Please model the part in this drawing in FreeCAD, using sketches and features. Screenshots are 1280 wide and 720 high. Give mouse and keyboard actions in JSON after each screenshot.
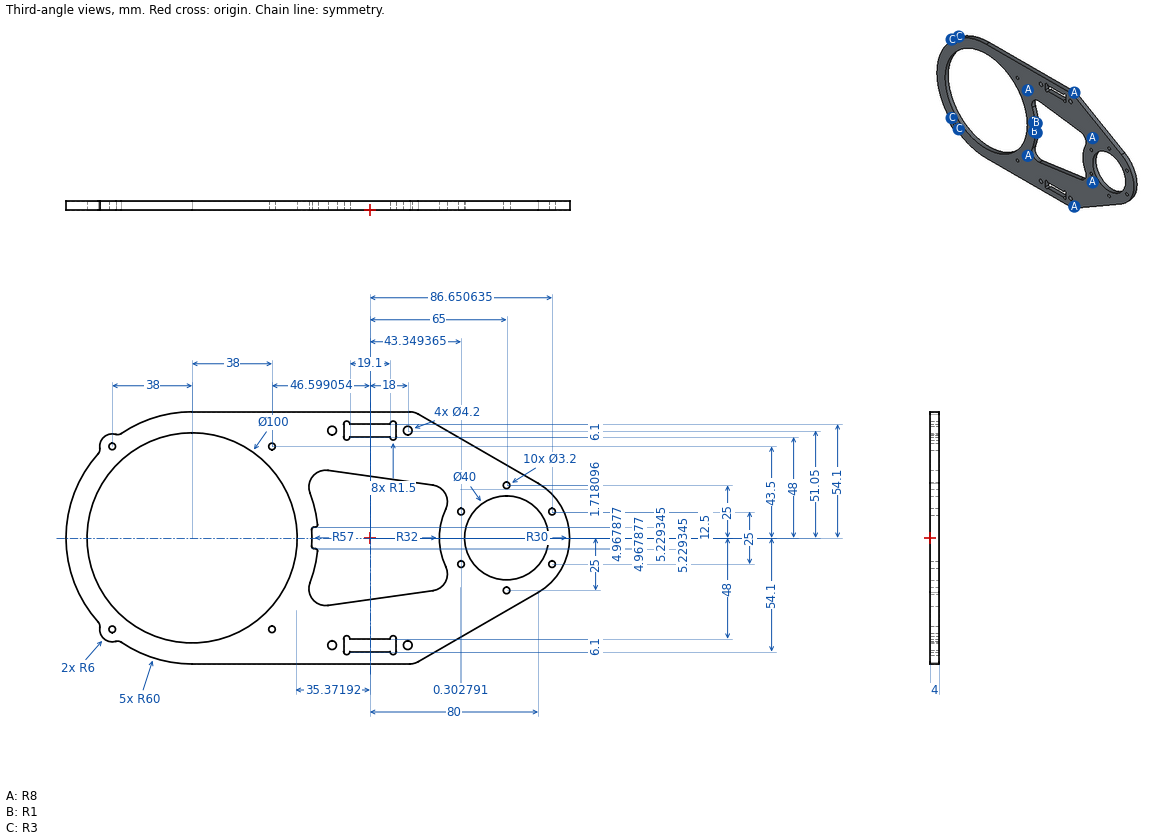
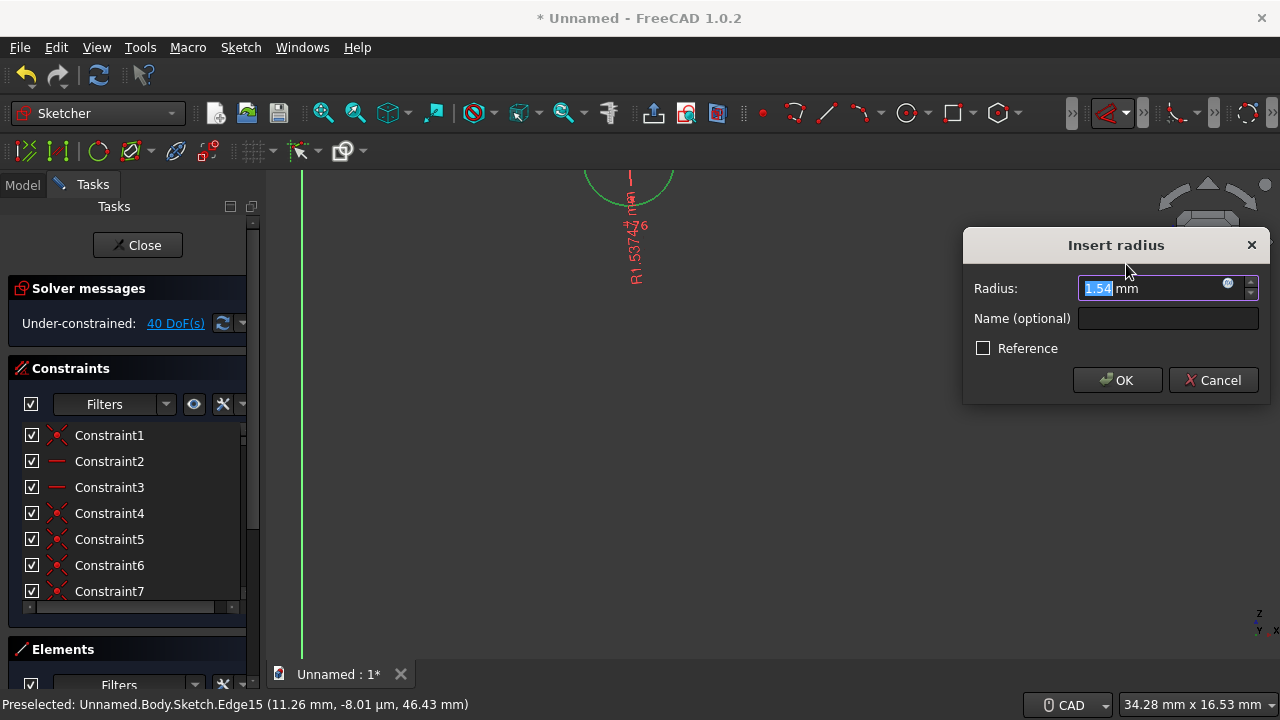
{"action": "type", "text": "1.5"}
{"action": "key", "text": "Return"}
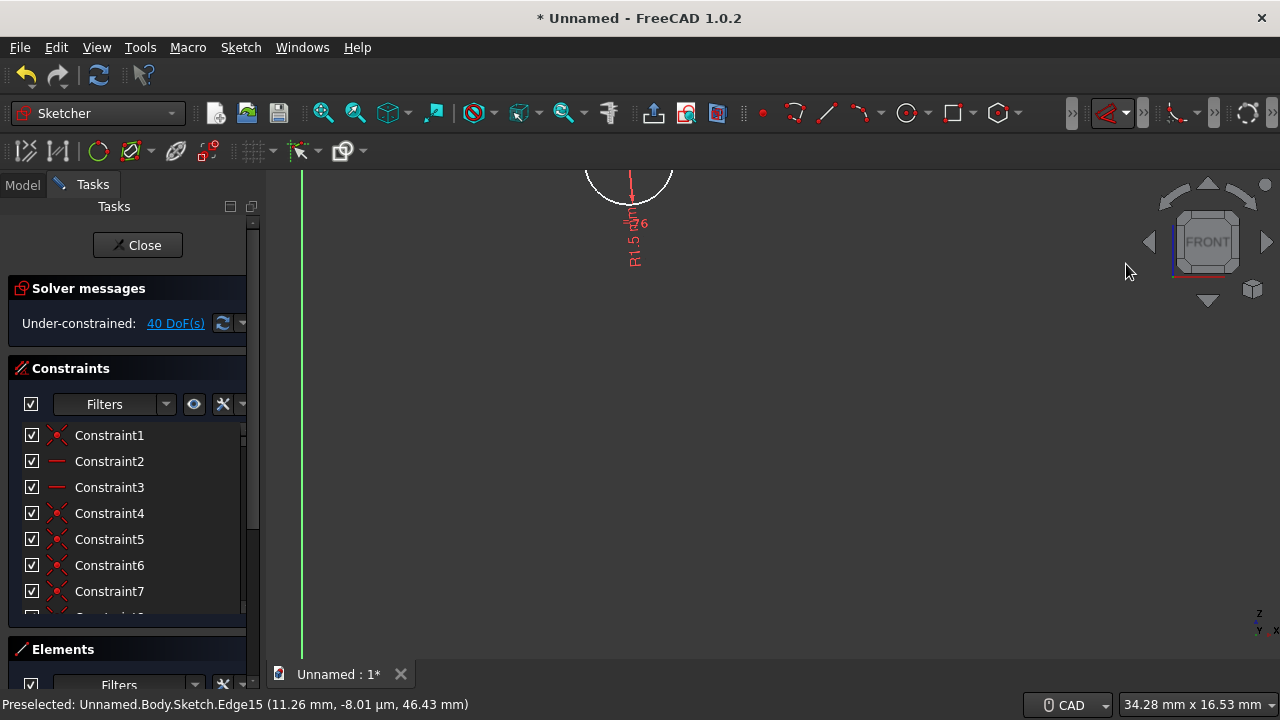
{"action": "scroll", "coordinate": [796, 321], "scroll_direction": "down", "scroll_amount": 13}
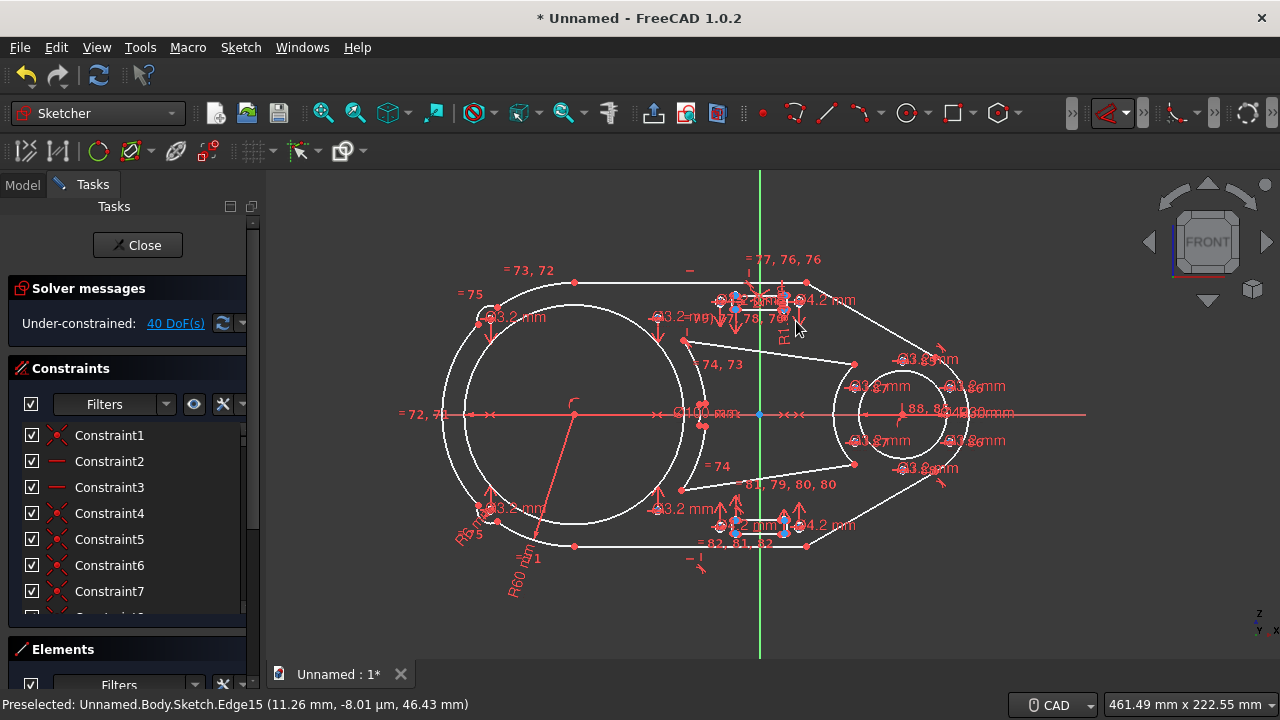
{"action": "left_click", "coordinate": [837, 393]}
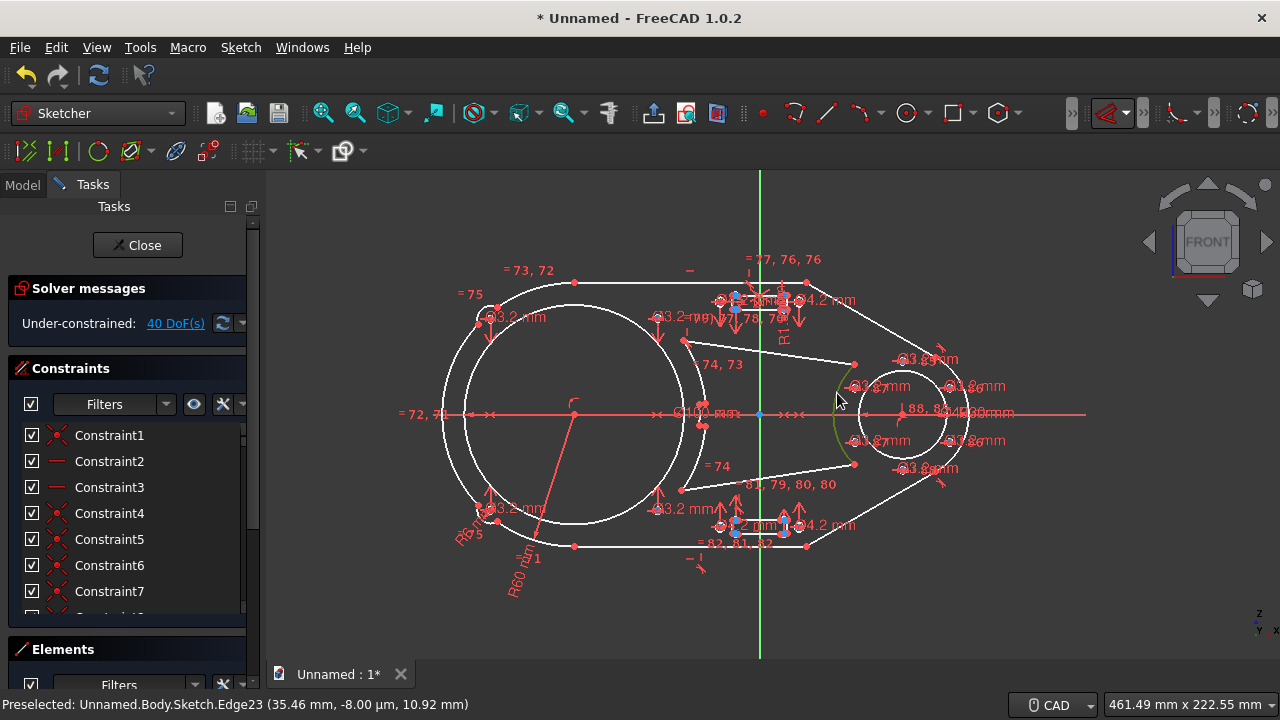
{"action": "left_click", "coordinate": [1128, 114]}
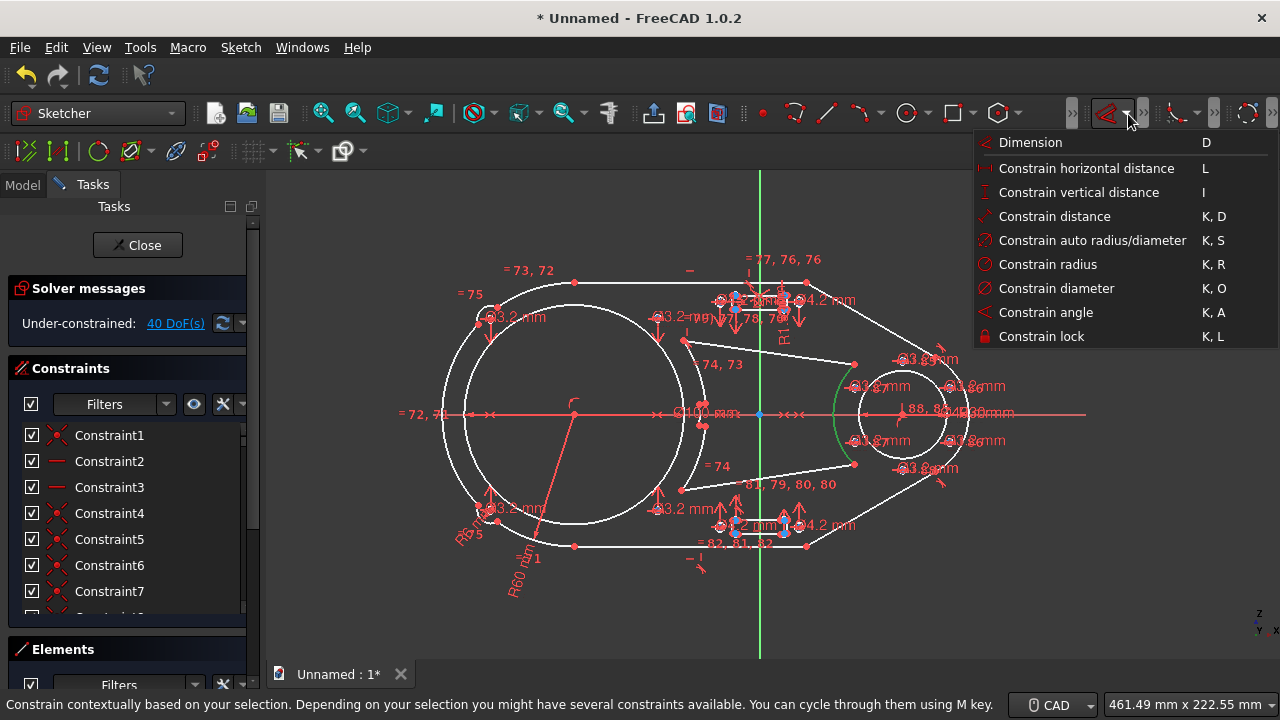
{"action": "left_click", "coordinate": [1126, 264]}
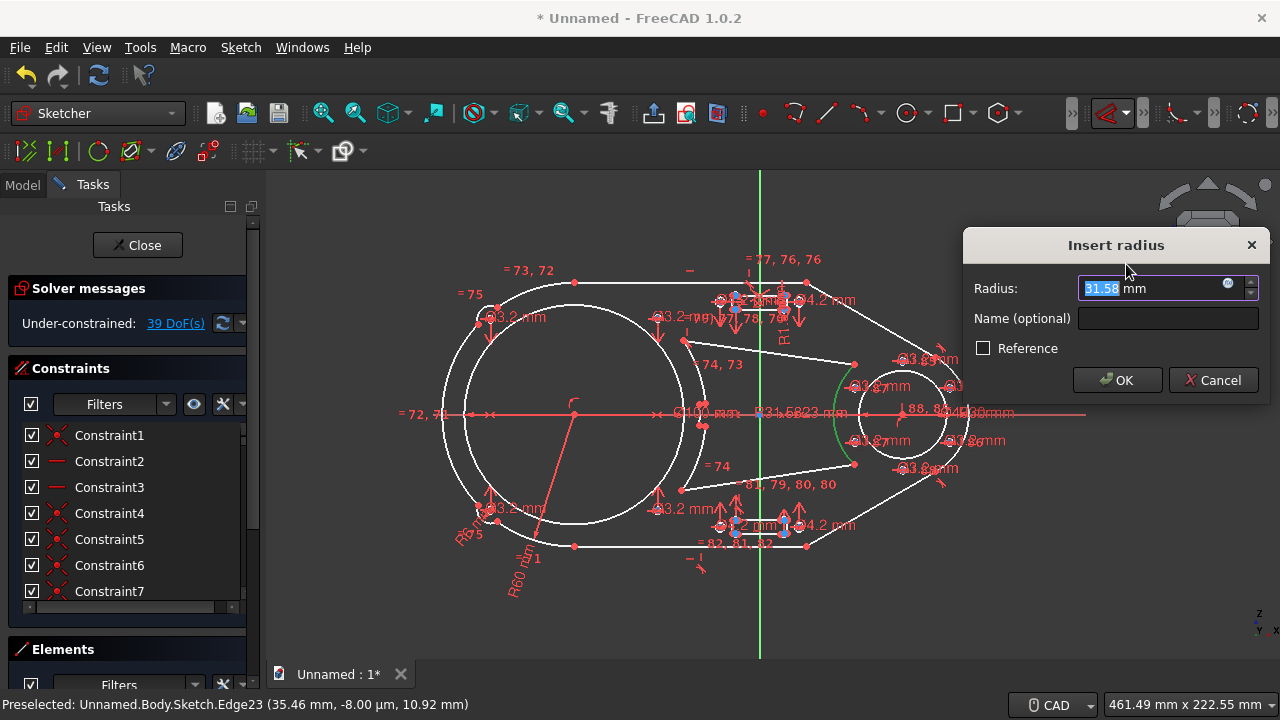
{"action": "type", "text": "32"}
{"action": "key", "text": "Return"}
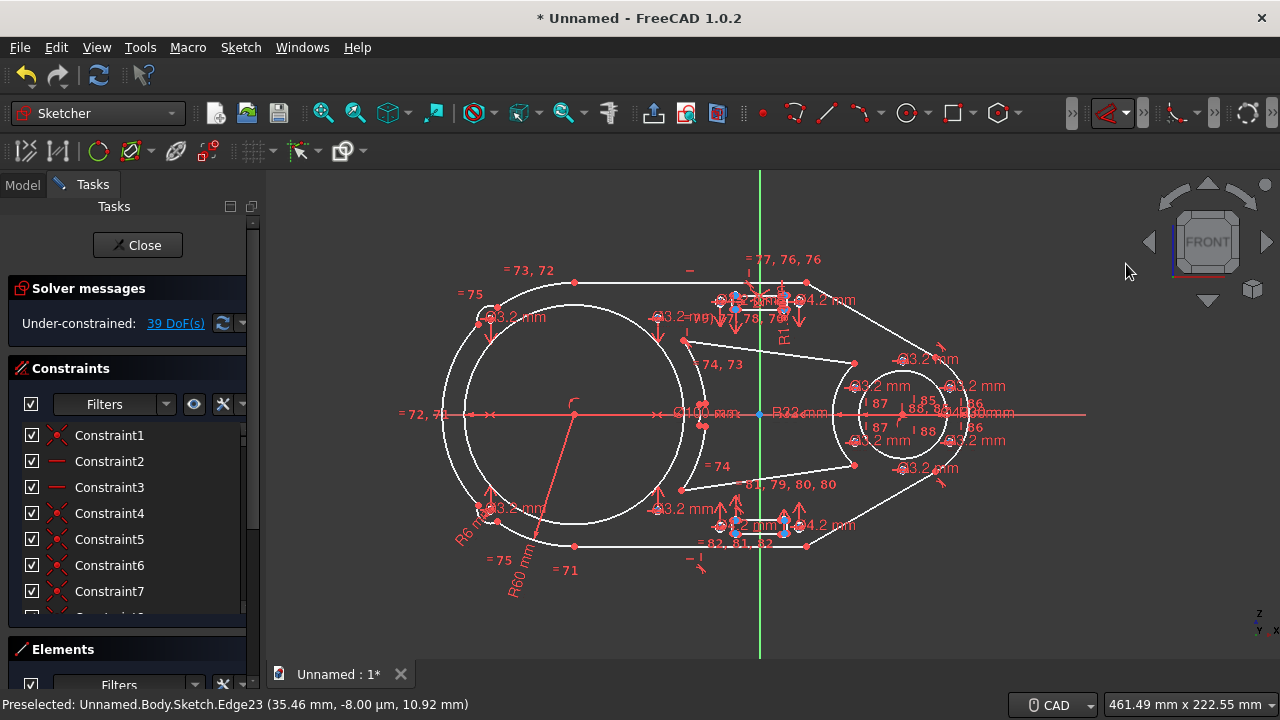
{"action": "scroll", "coordinate": [700, 415], "scroll_direction": "up", "scroll_amount": 2}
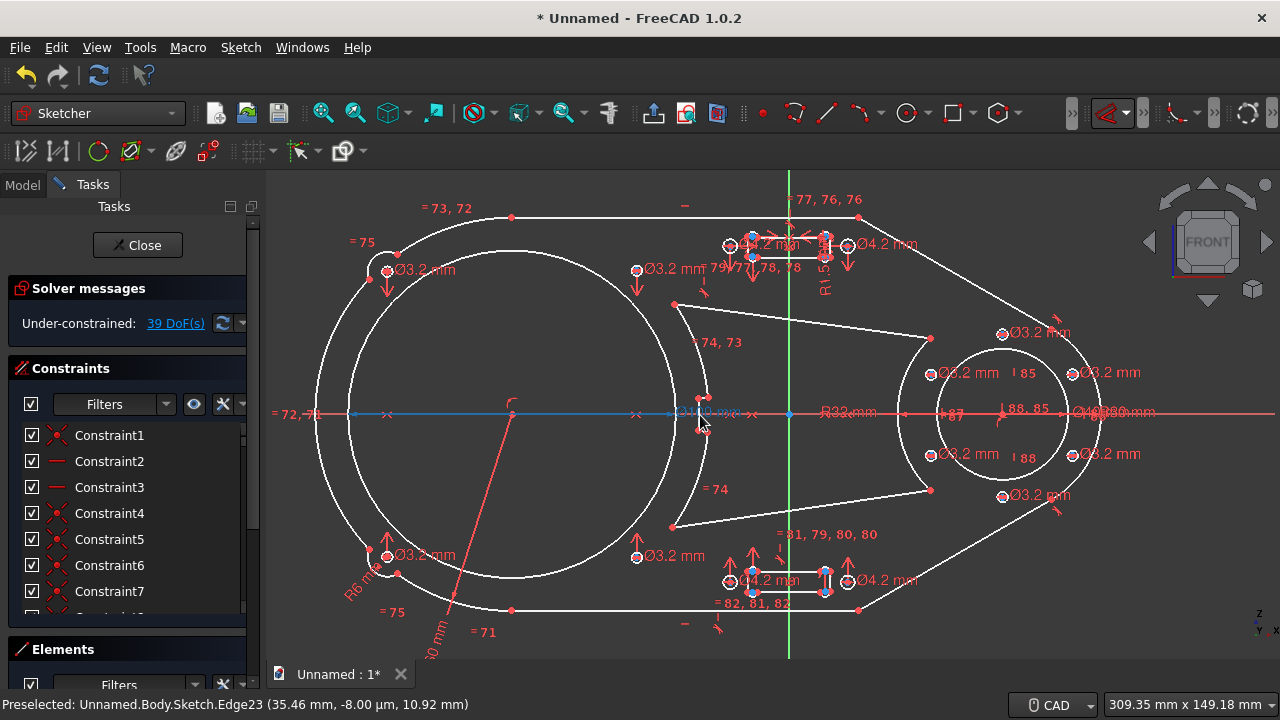
{"action": "left_click", "coordinate": [699, 421]}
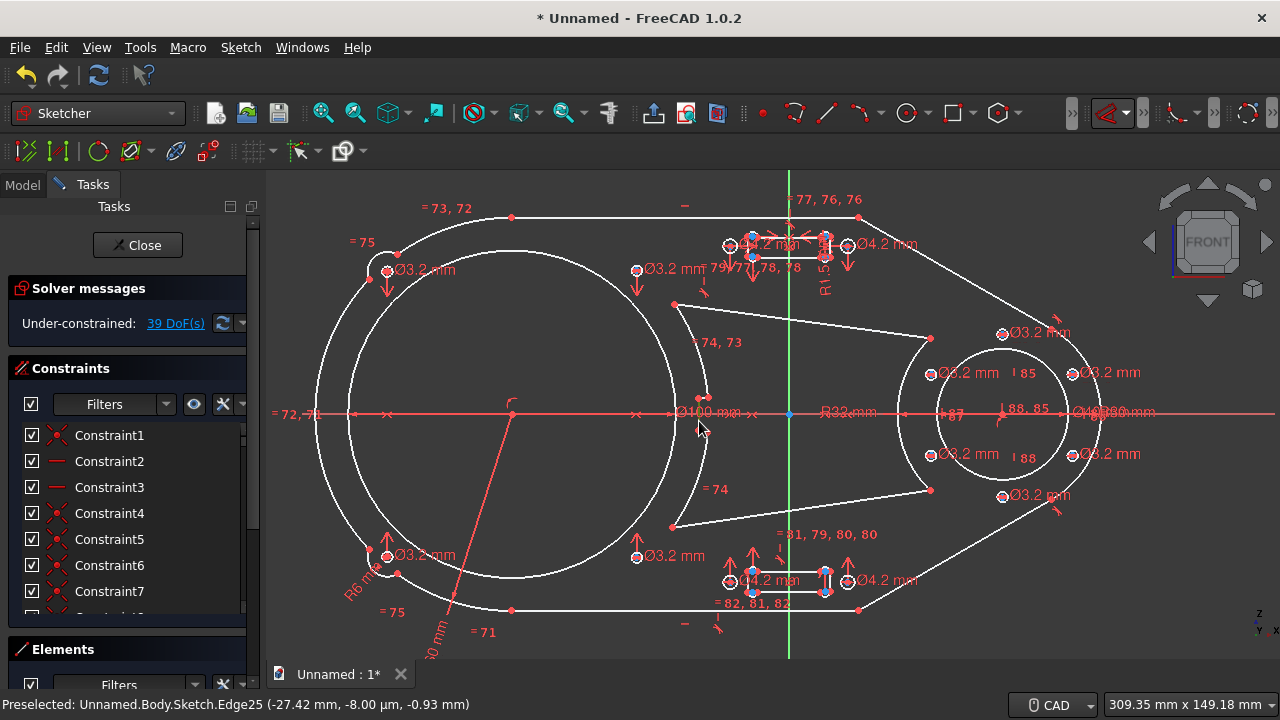
{"action": "key", "text": "k r"}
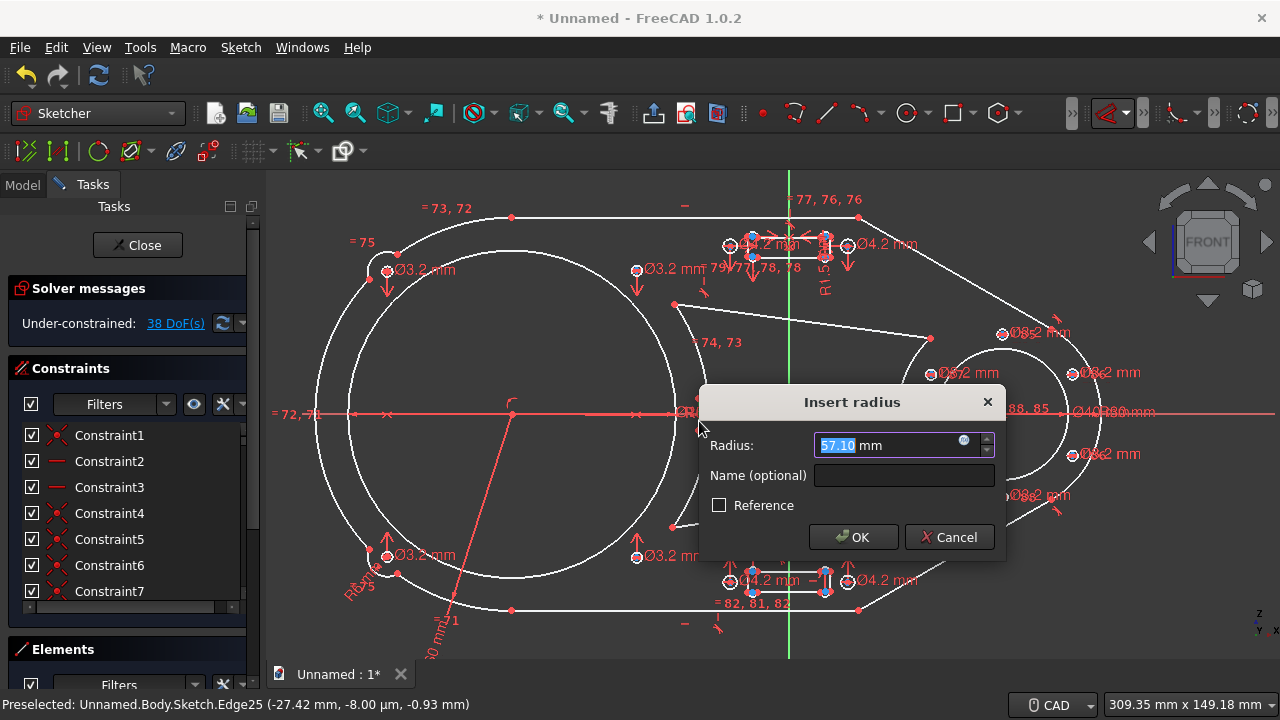
{"action": "type", "text": "57"}
{"action": "key", "text": "Return"}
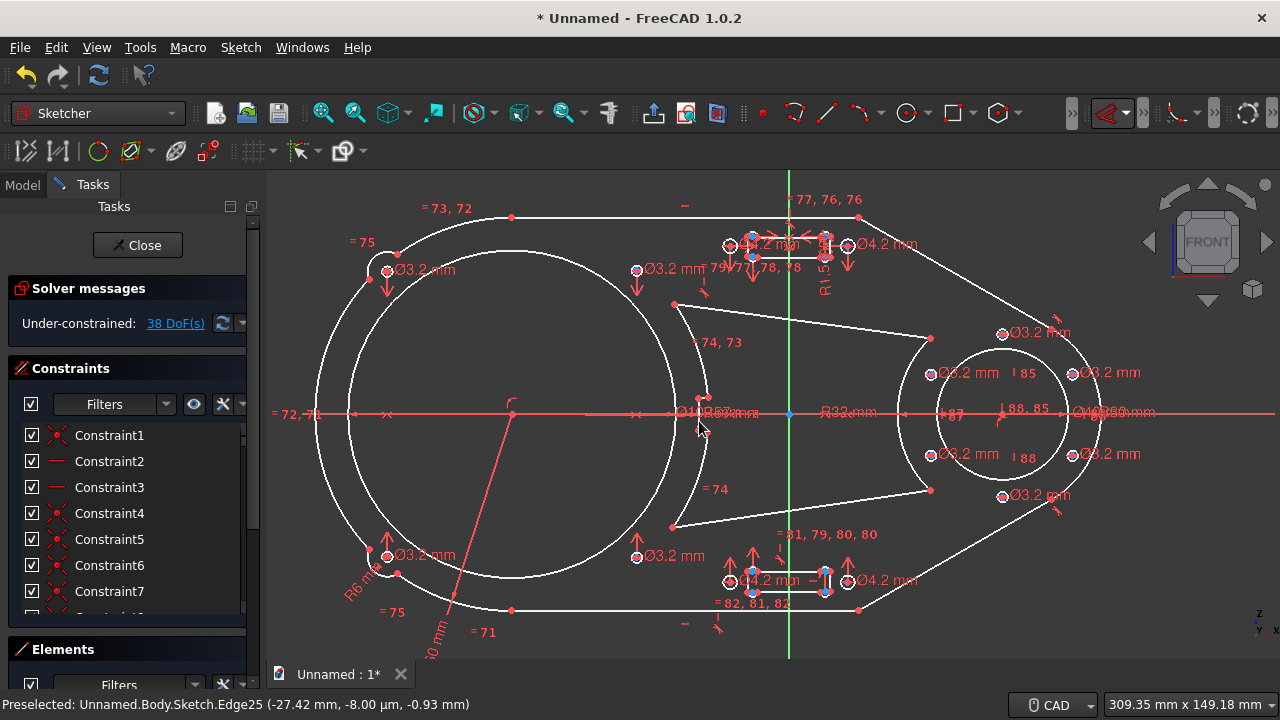
{"action": "left_click", "coordinate": [848, 246]}